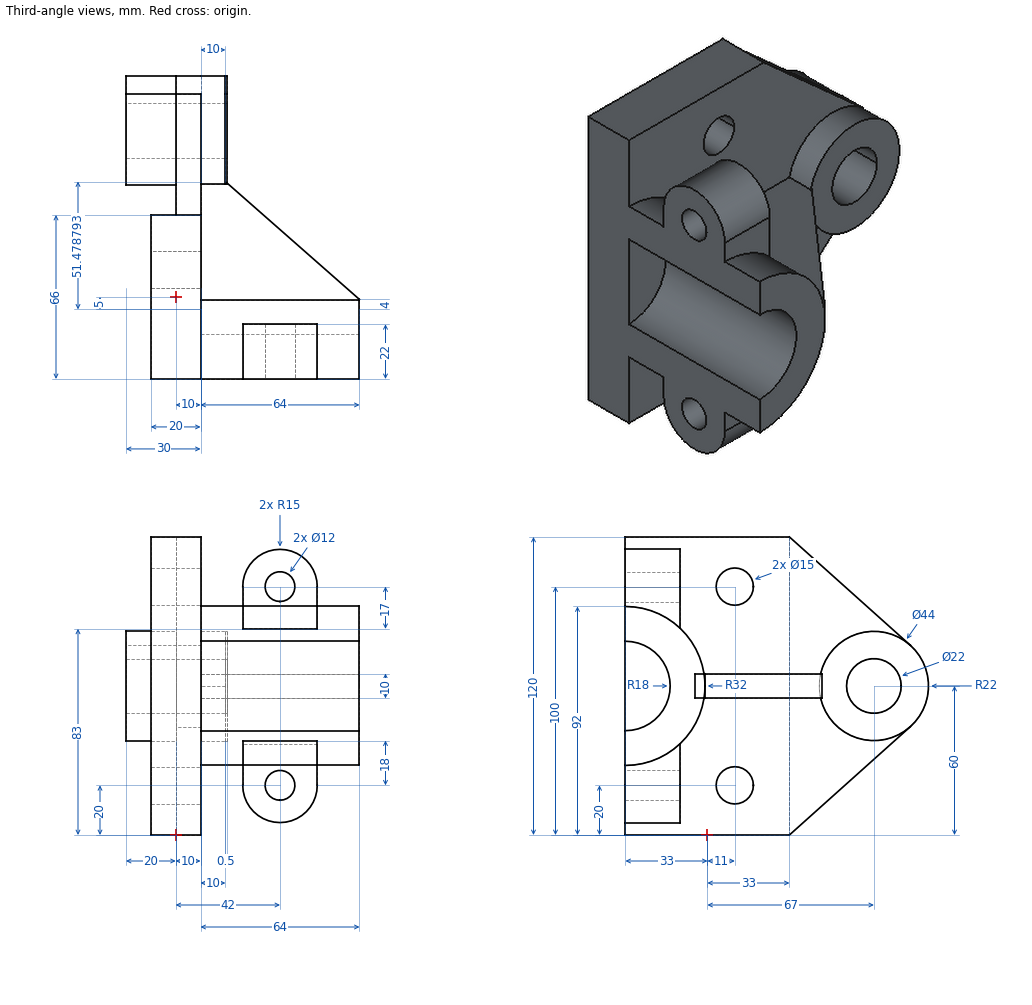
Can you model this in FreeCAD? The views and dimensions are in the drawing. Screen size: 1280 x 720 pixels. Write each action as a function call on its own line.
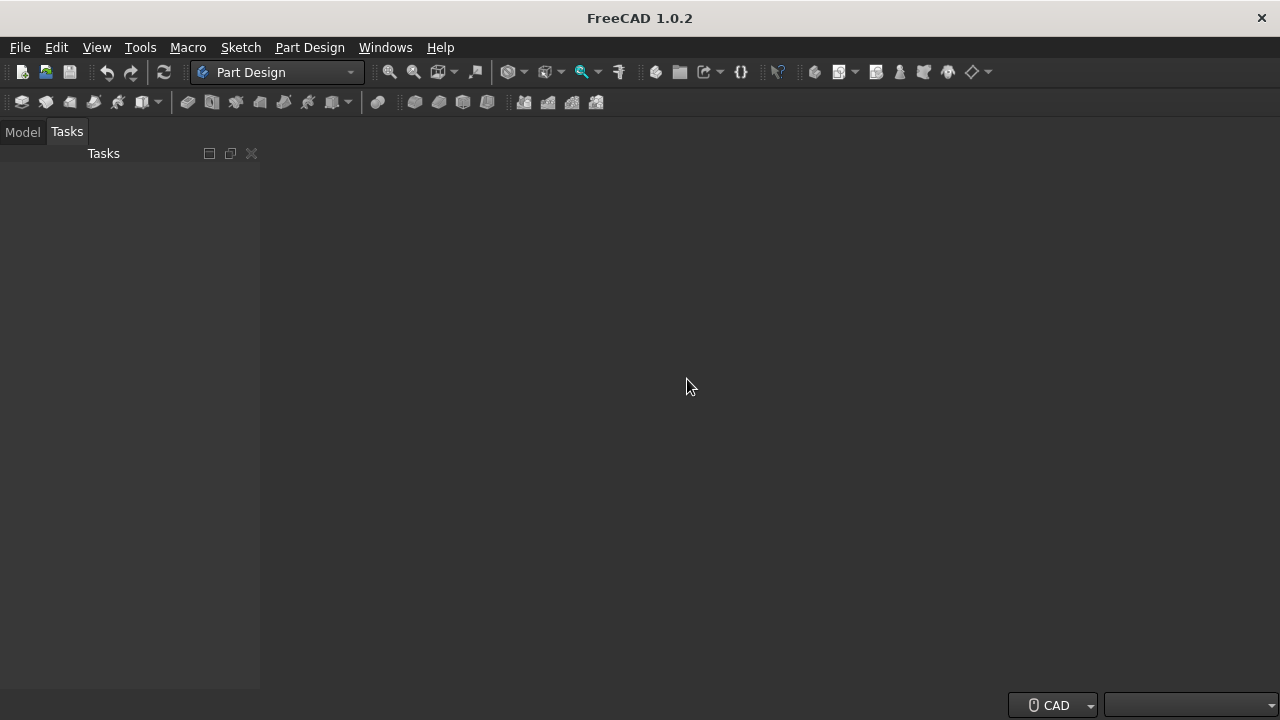
click(22, 72)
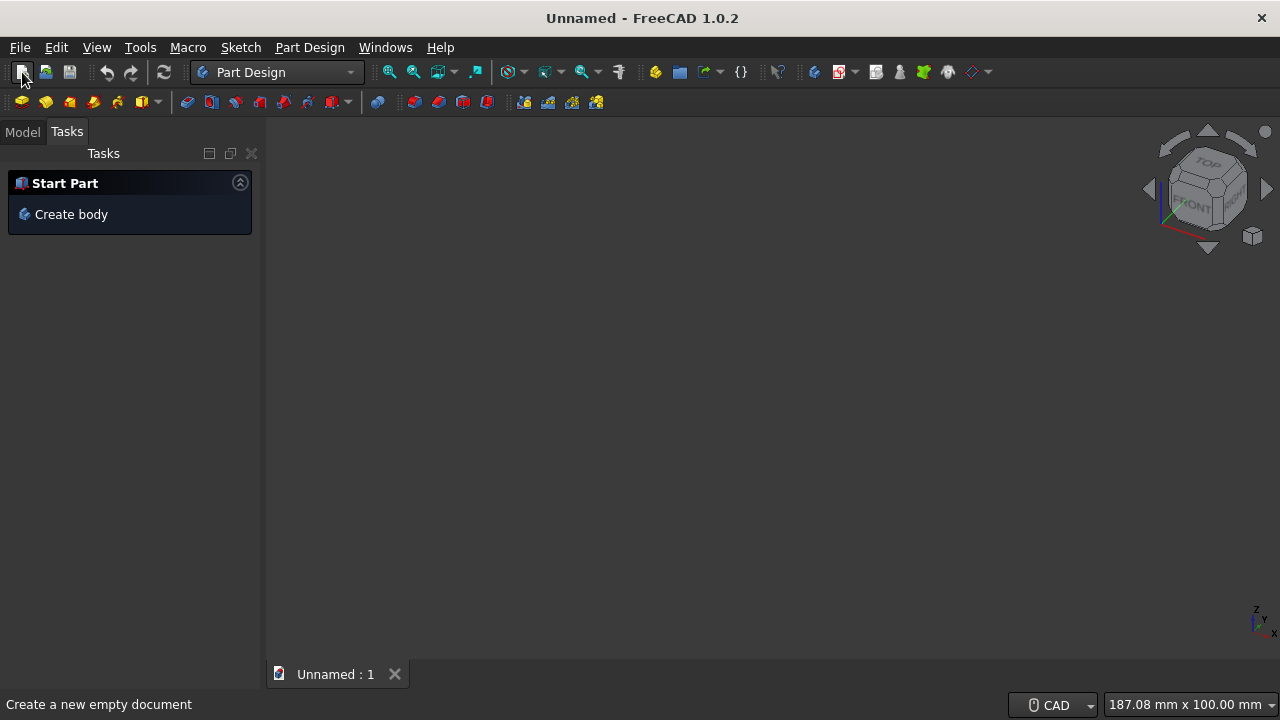
click(840, 72)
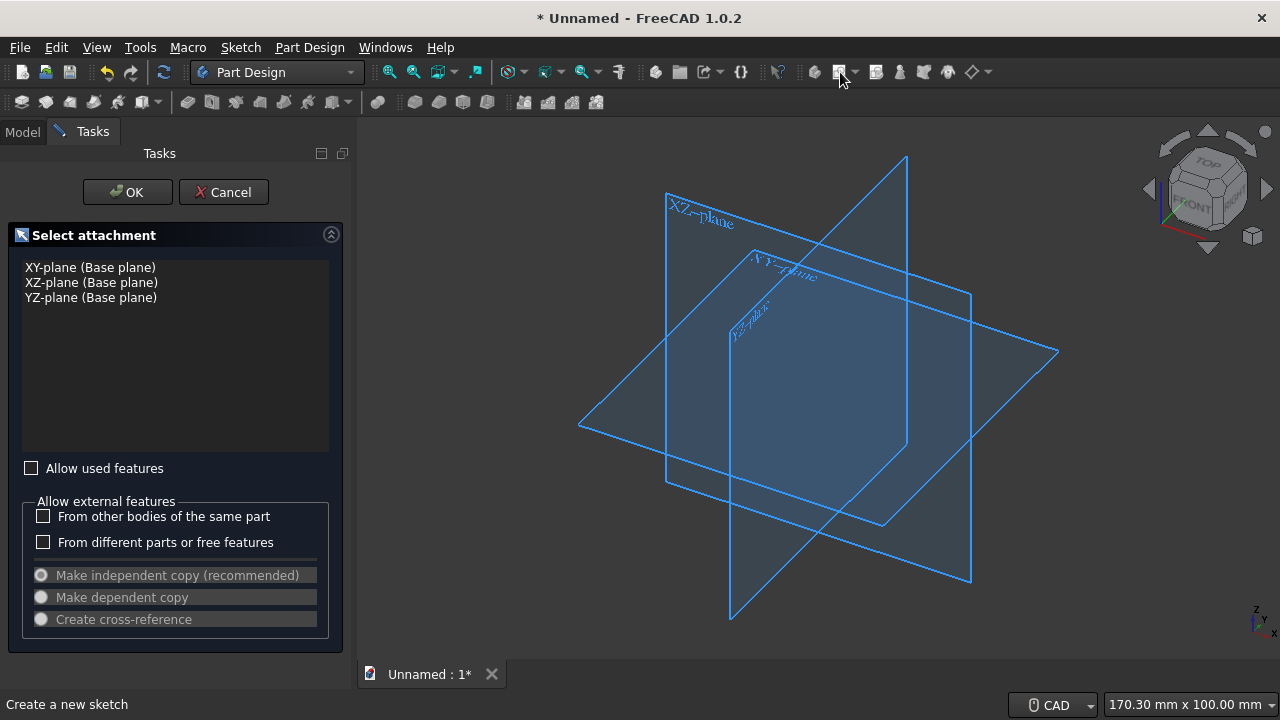
click(82, 268)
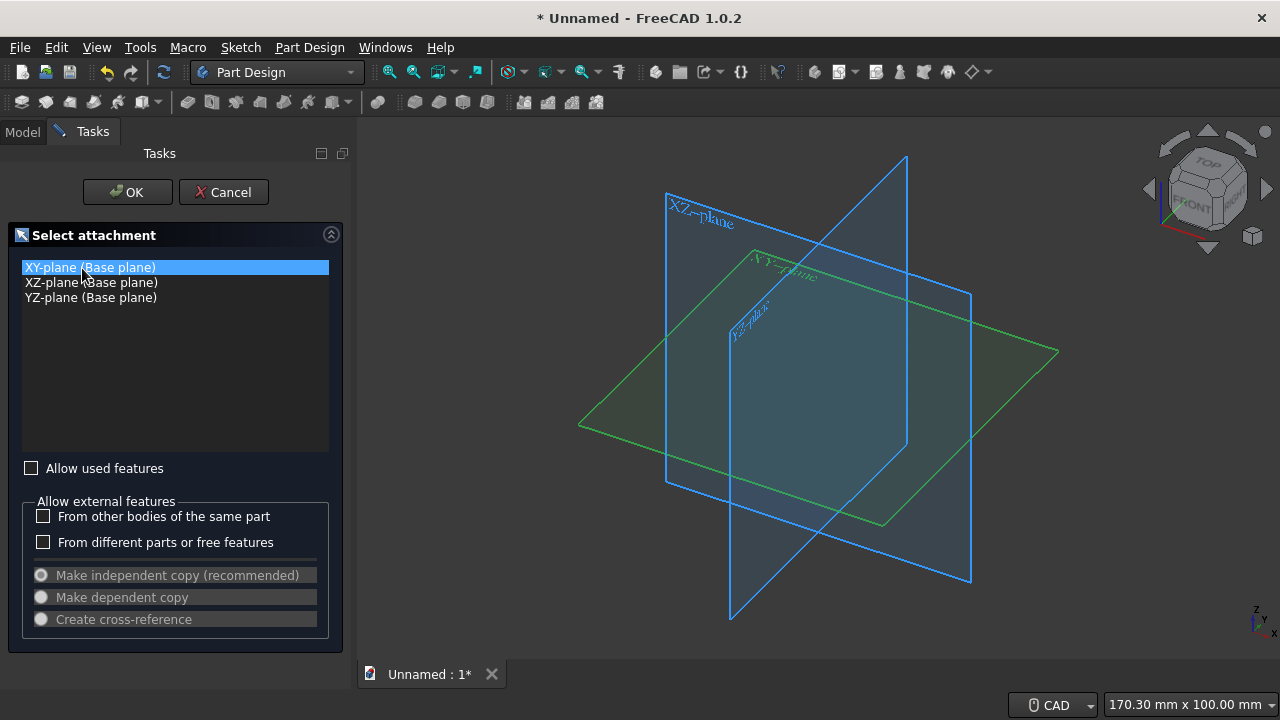
click(128, 192)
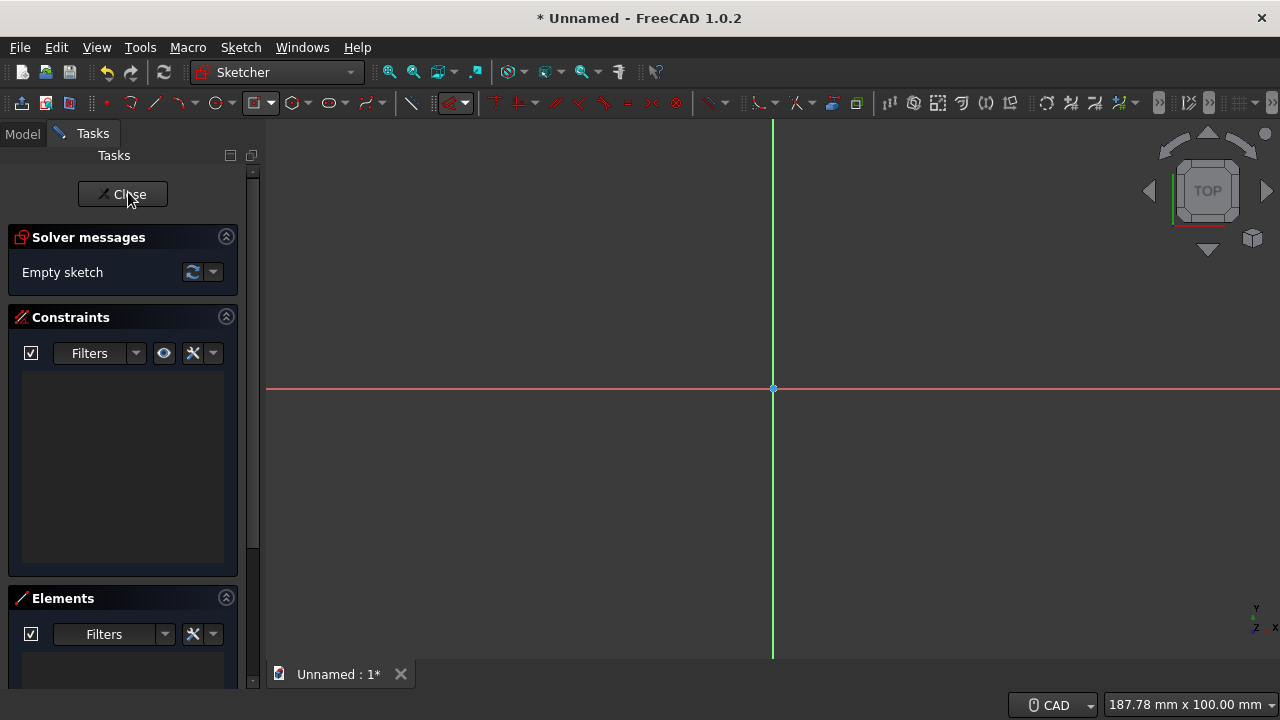
click(254, 104)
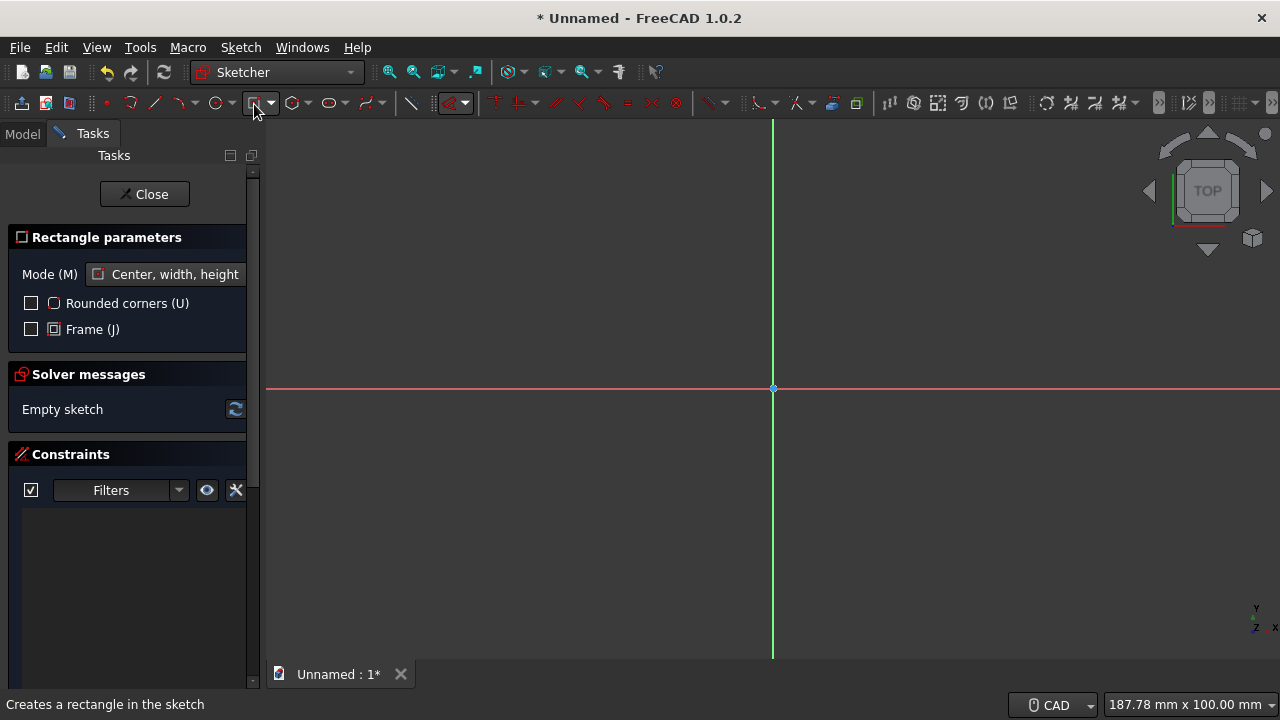
click(773, 389)
click(827, 211)
key(Escape)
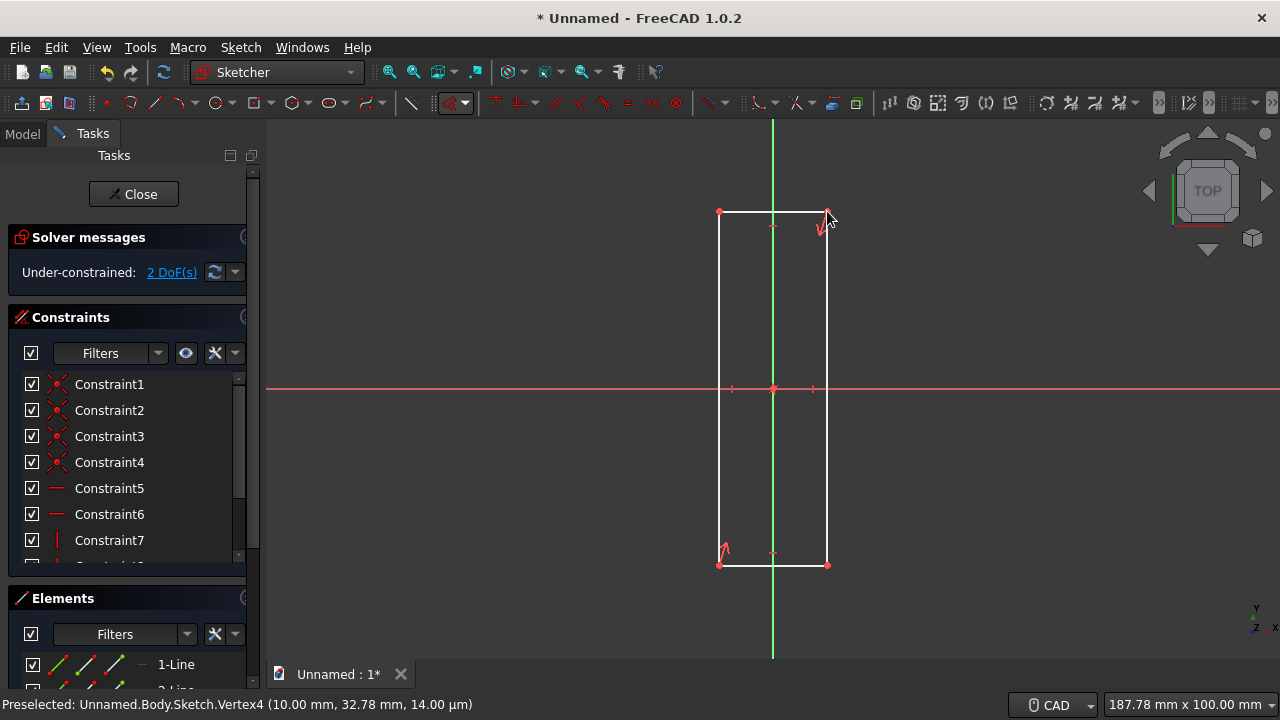
click(450, 104)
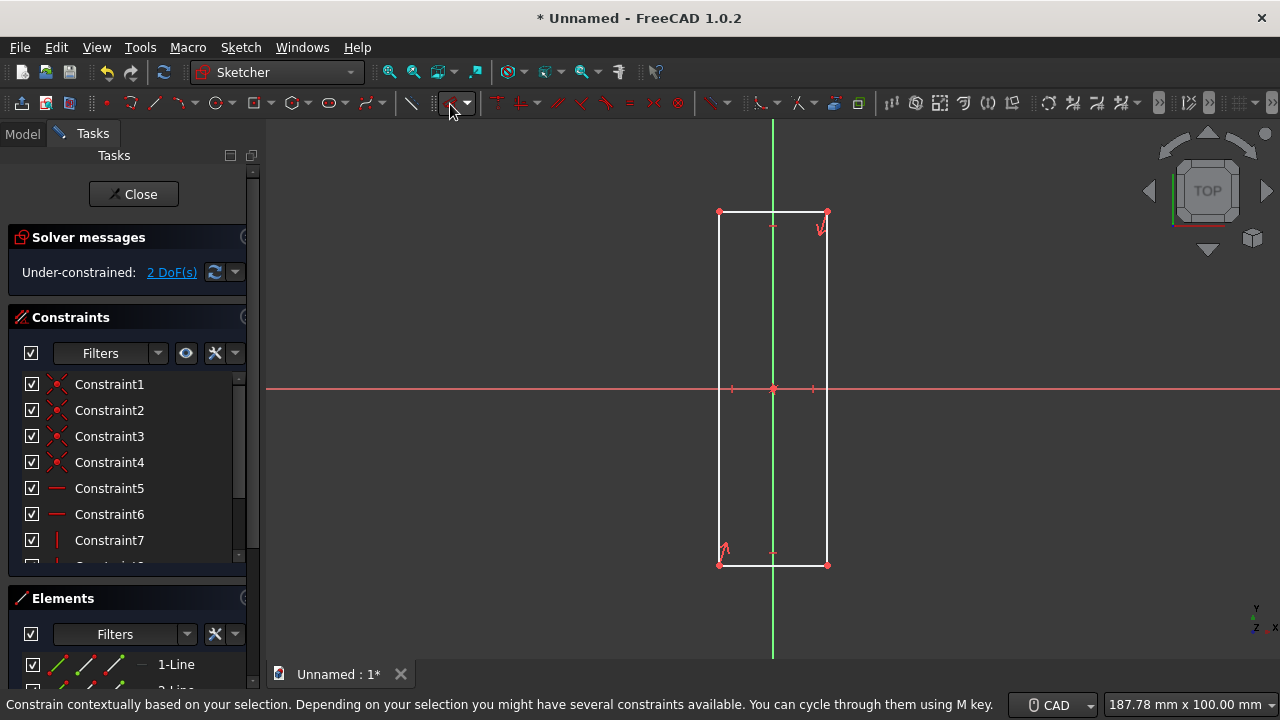
click(751, 566)
click(748, 600)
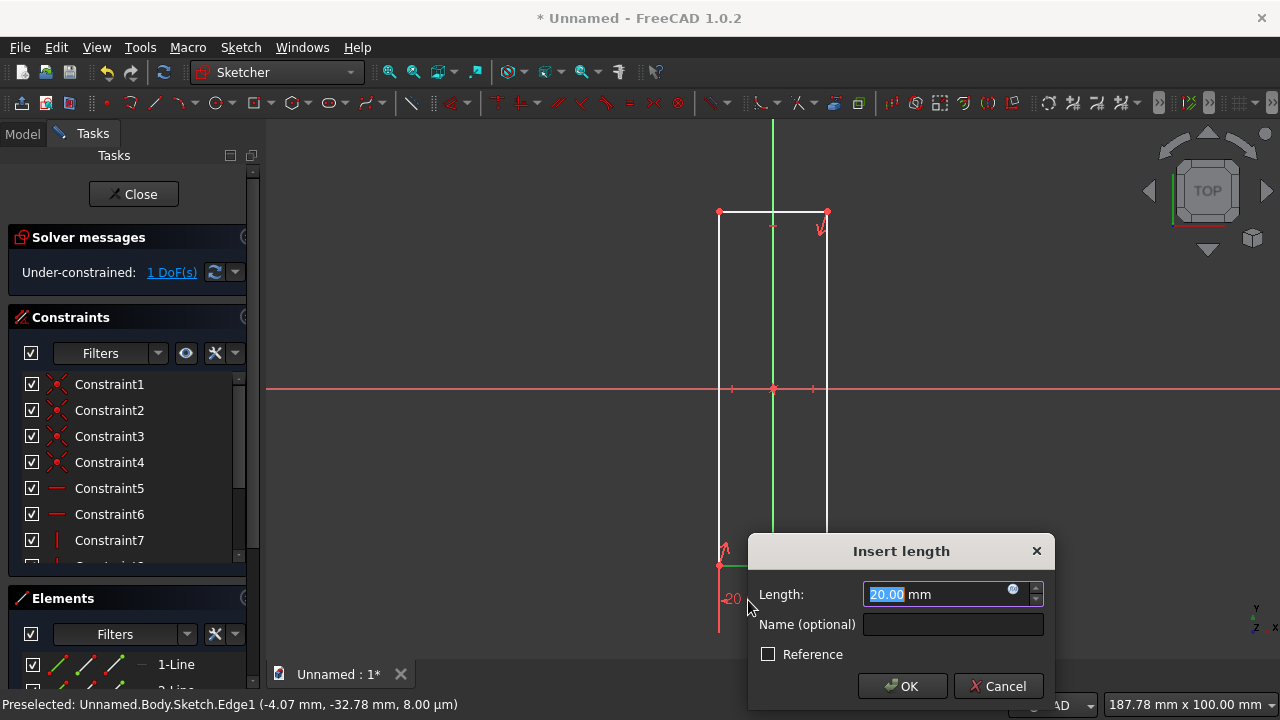
text(20)
key(Return)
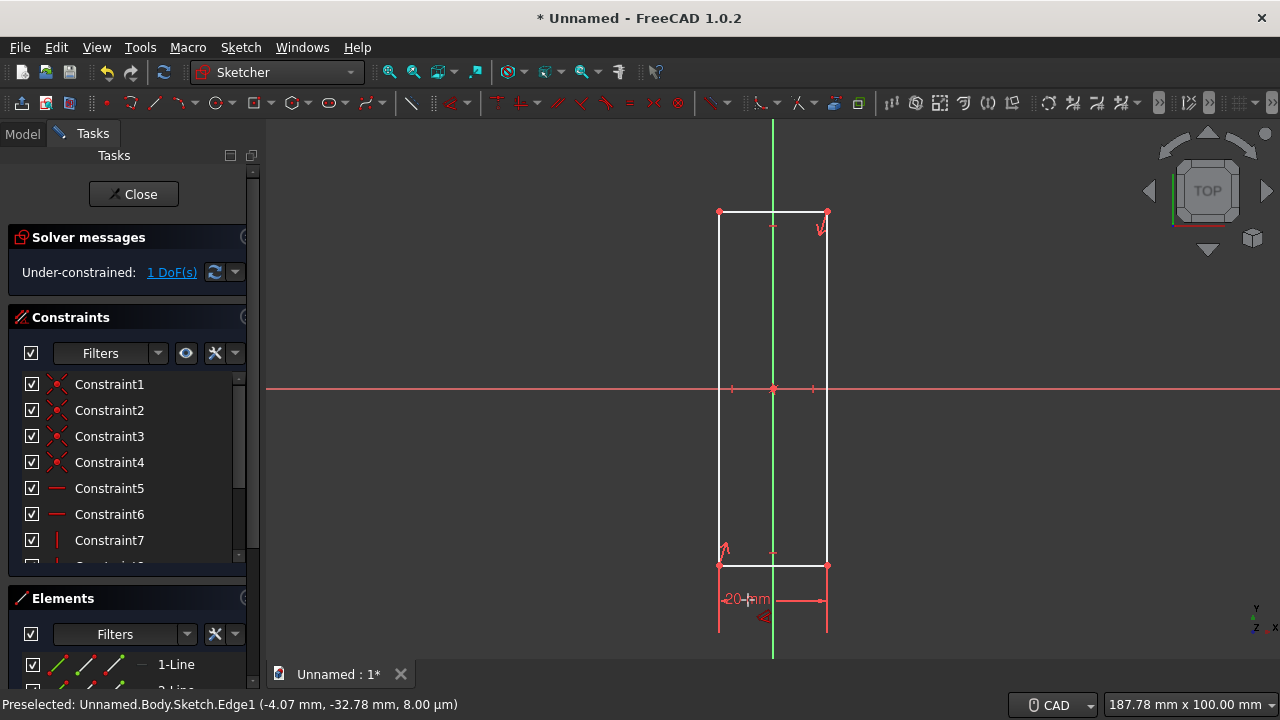
click(827, 460)
click(861, 308)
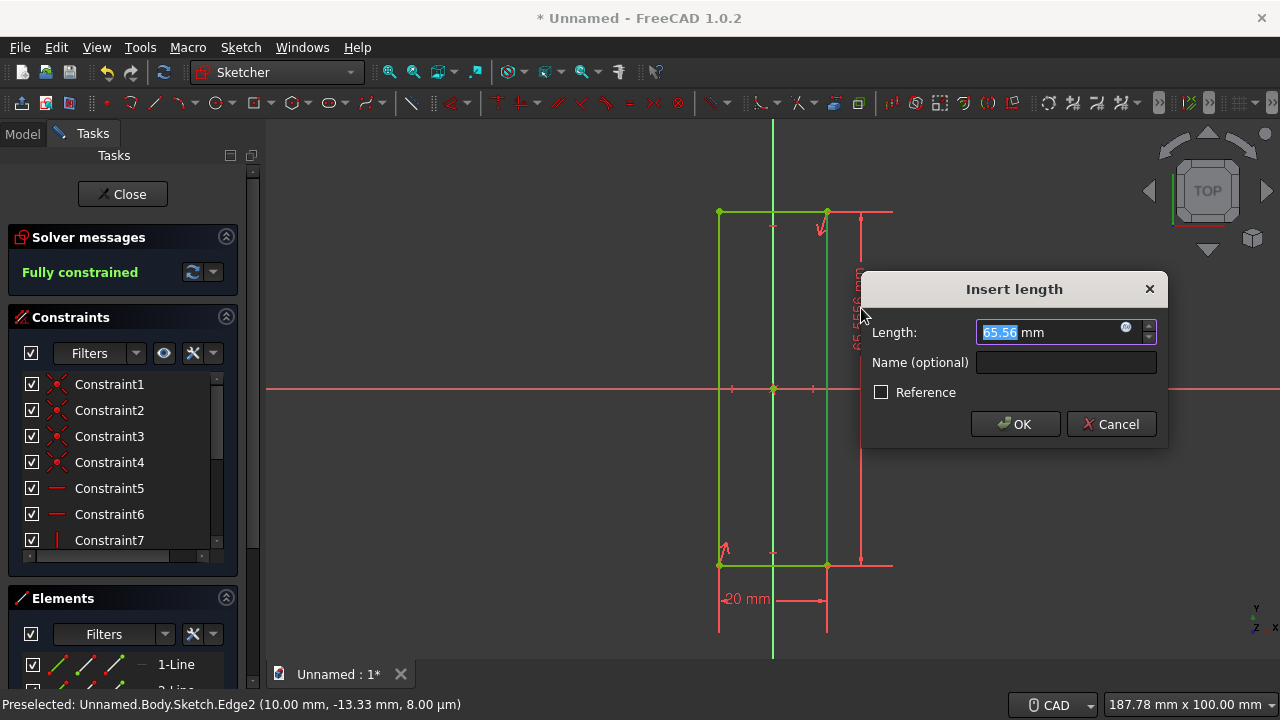
text(66)
key(Return)
key(Escape)